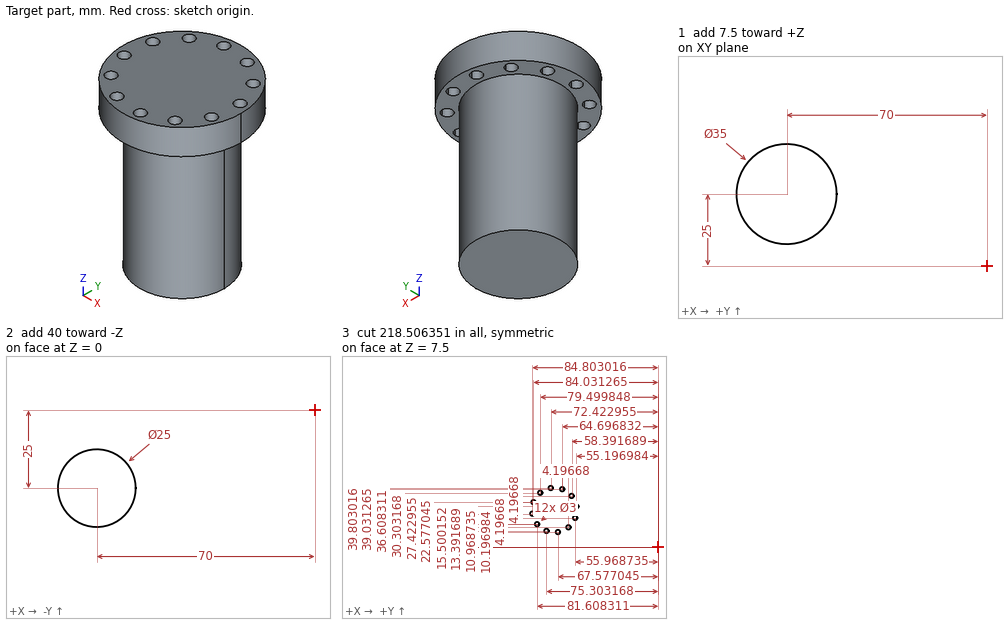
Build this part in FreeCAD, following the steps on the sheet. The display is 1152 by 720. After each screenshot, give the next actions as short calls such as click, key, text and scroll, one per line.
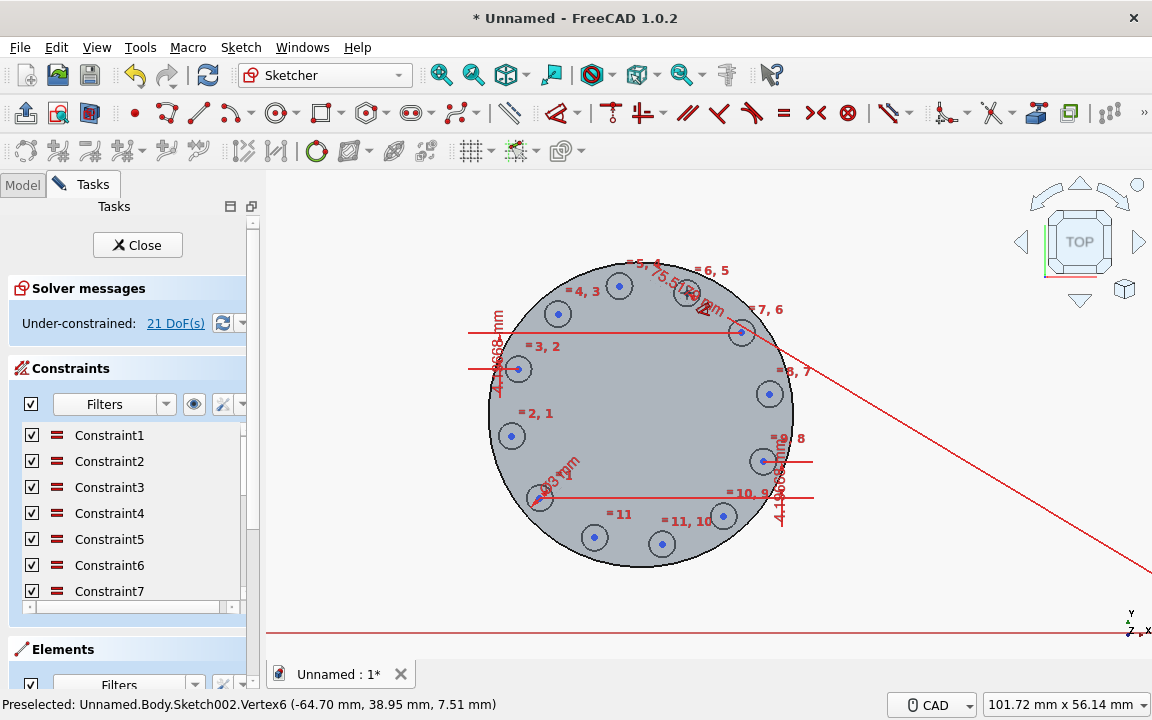
click(724, 516)
click(705, 259)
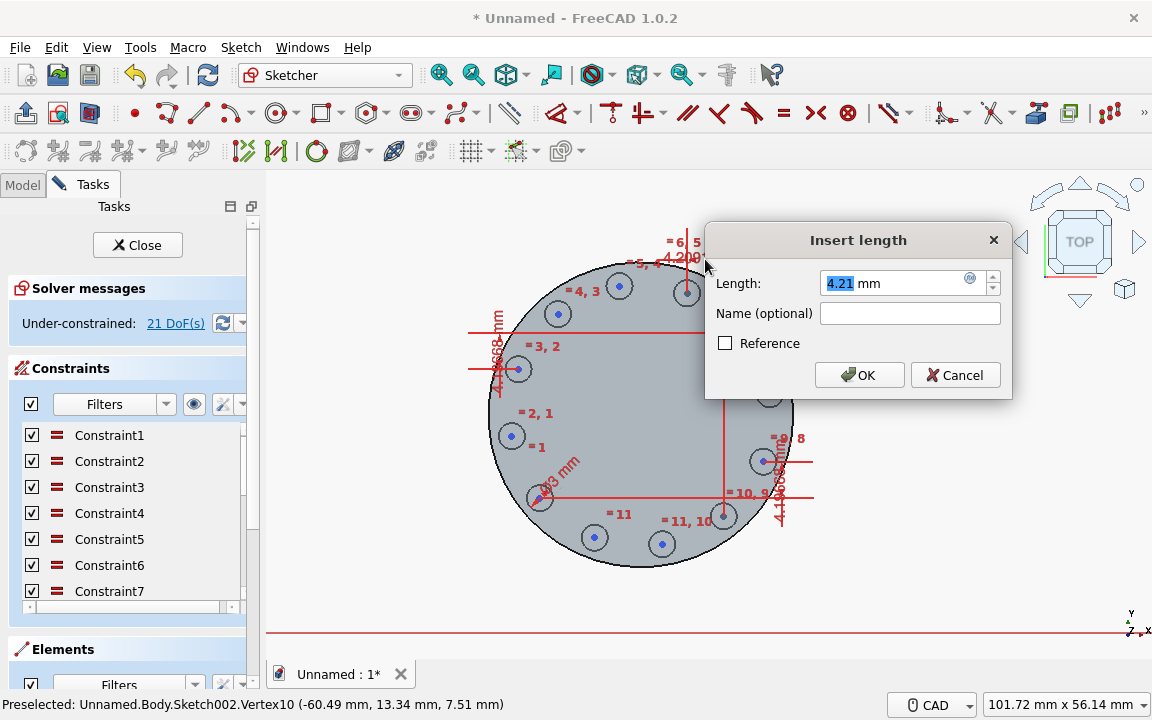
text(4.19668)
key(Return)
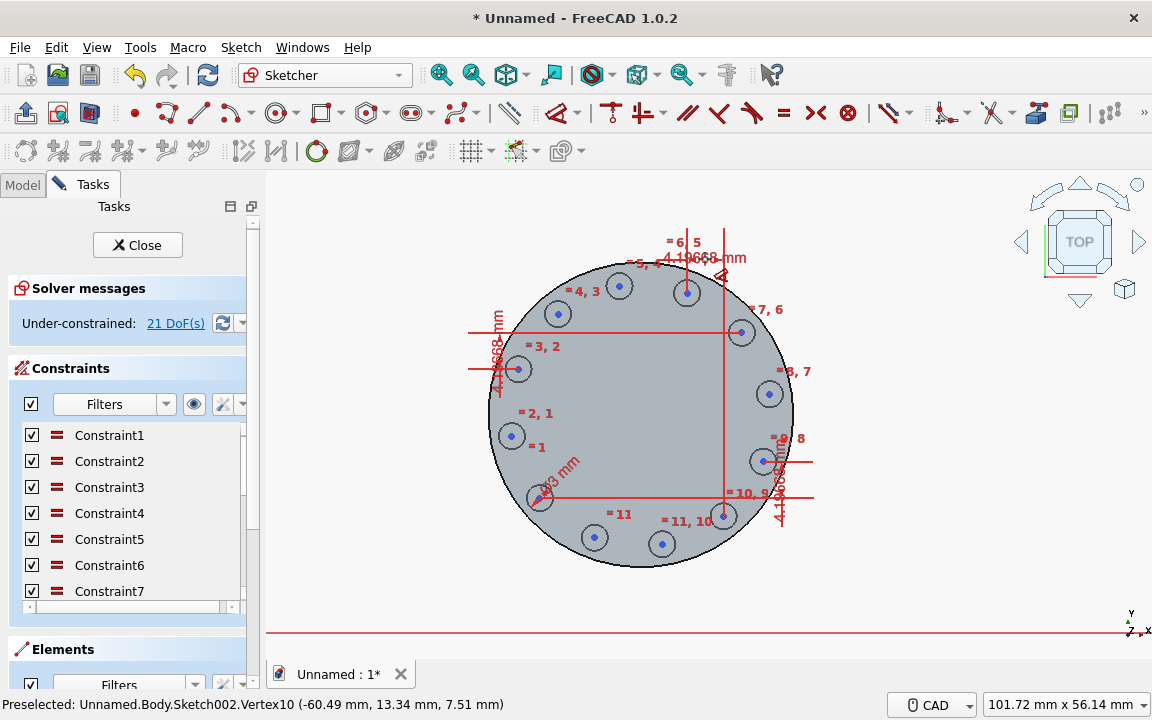
click(540, 498)
click(661, 464)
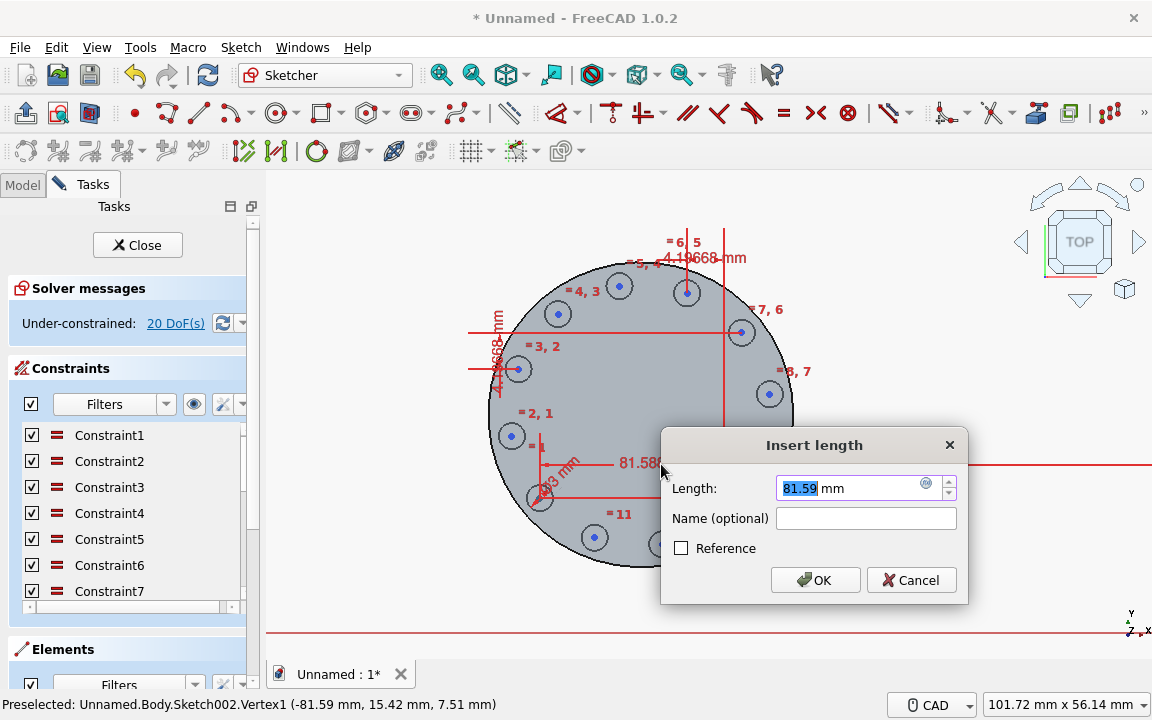
text(81.608311)
key(Return)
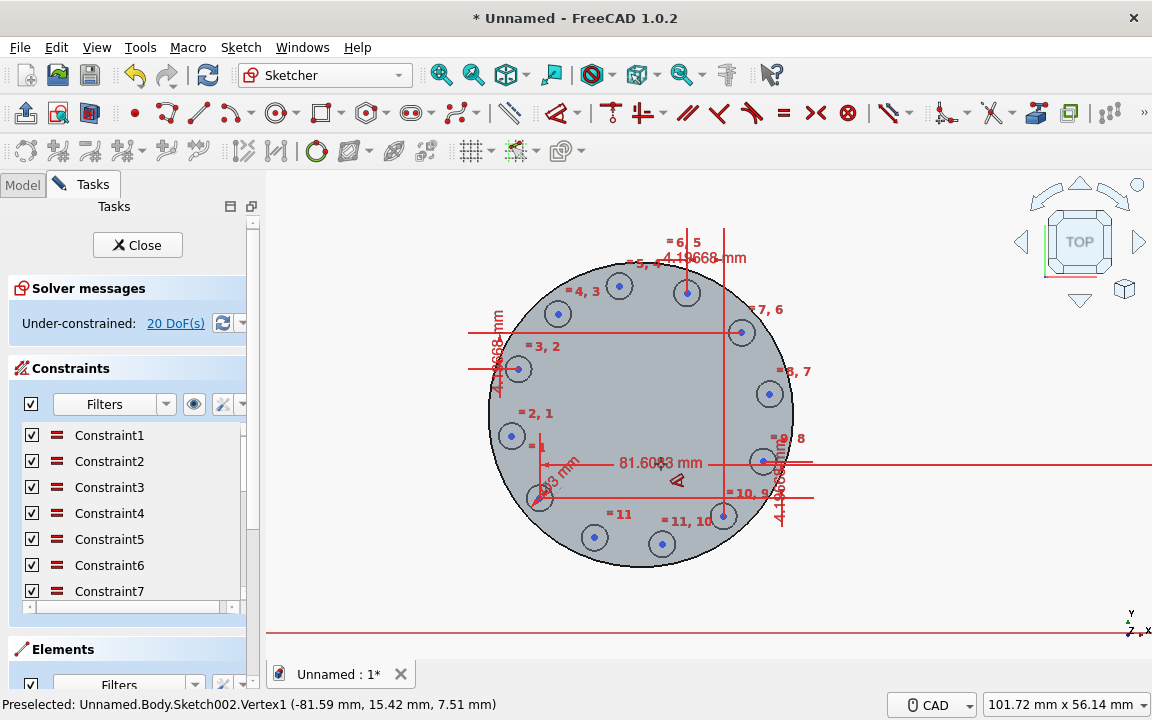
click(540, 498)
click(506, 565)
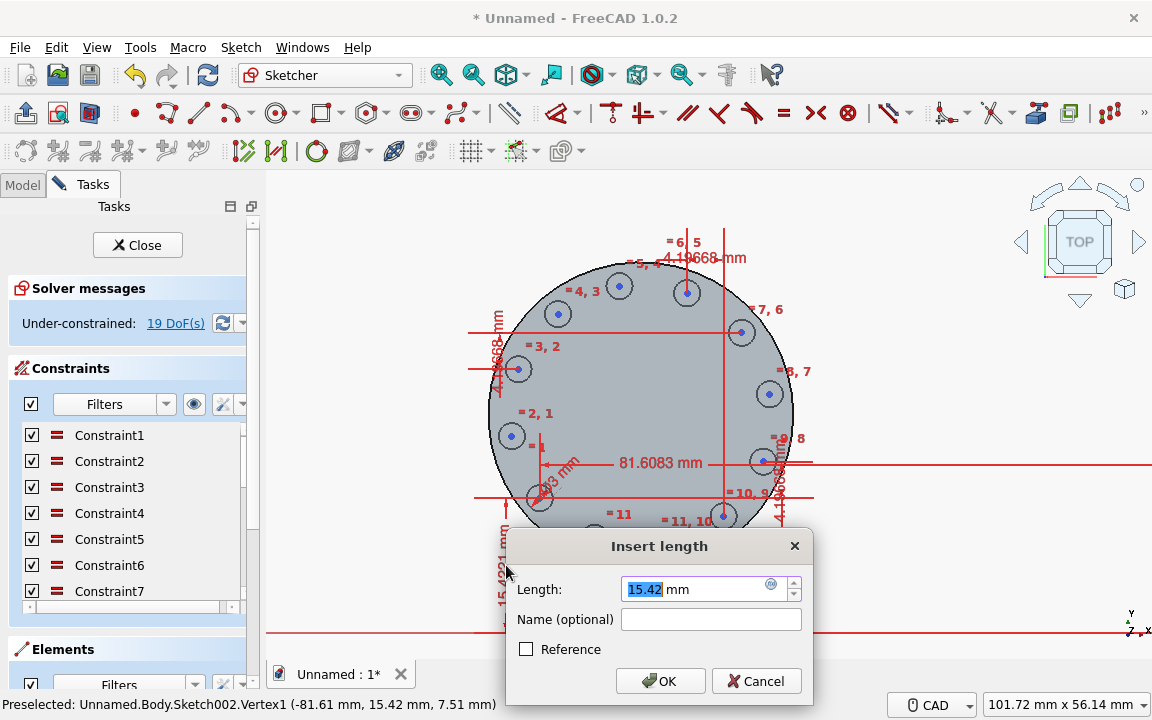
text(15.500152)
key(Return)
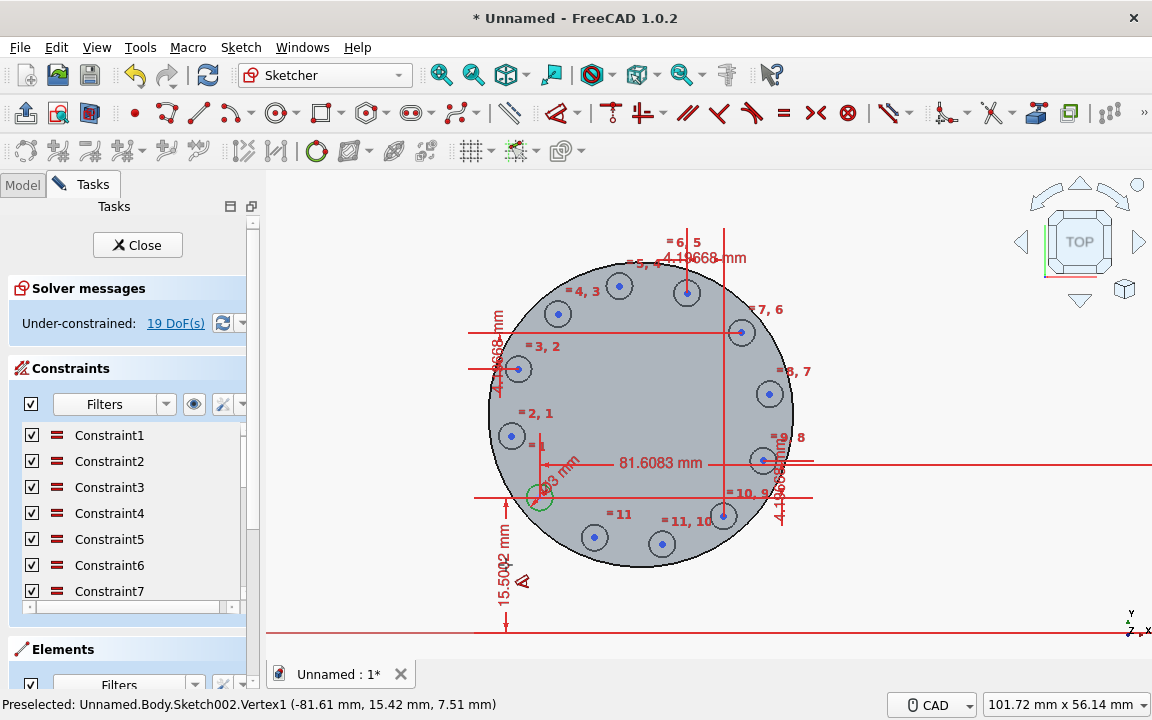
click(512, 436)
click(640, 402)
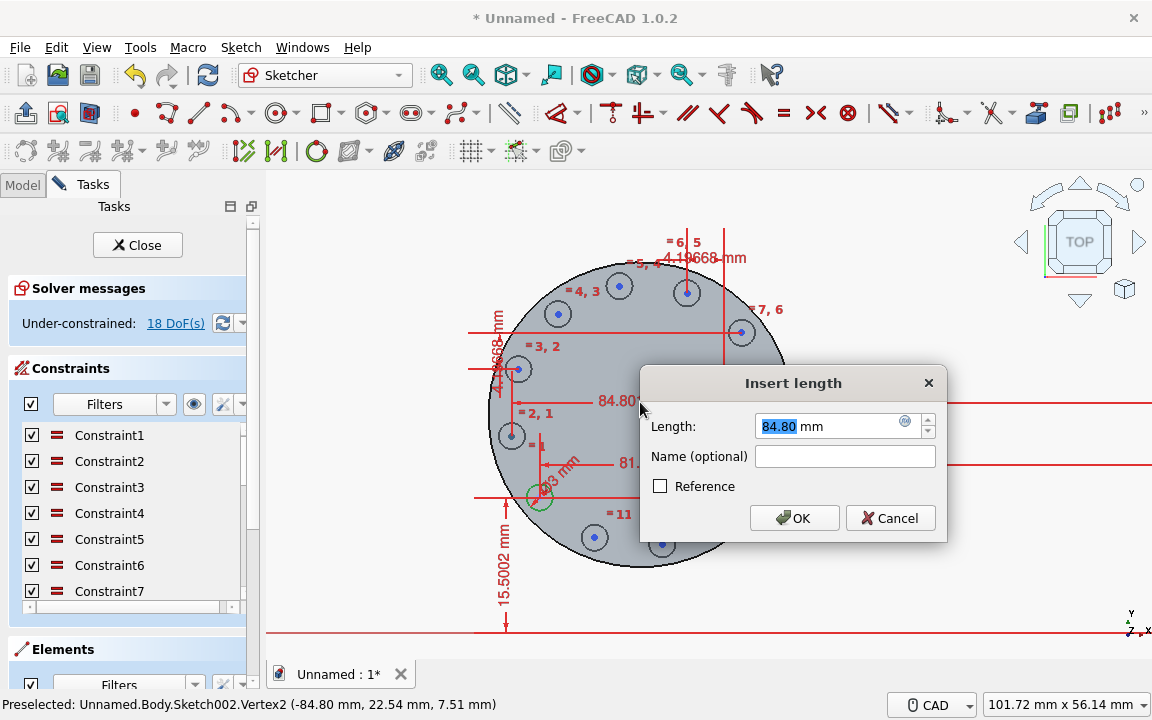
text(84.803016)
key(Return)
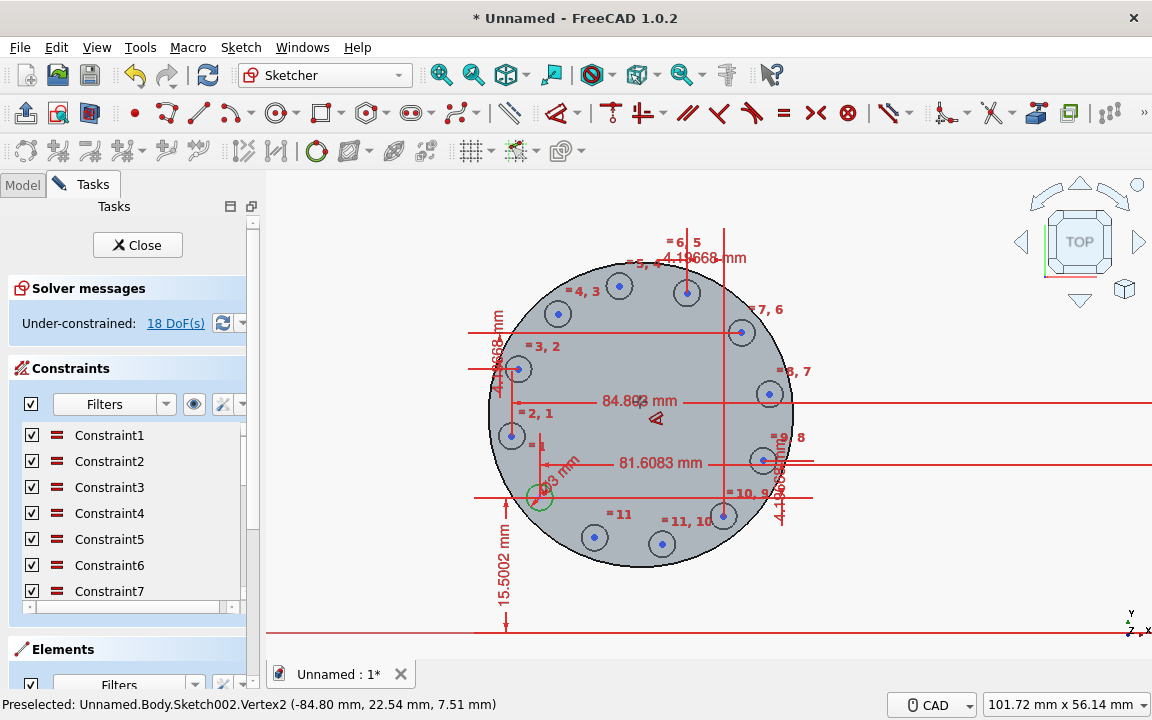
click(512, 436)
click(478, 534)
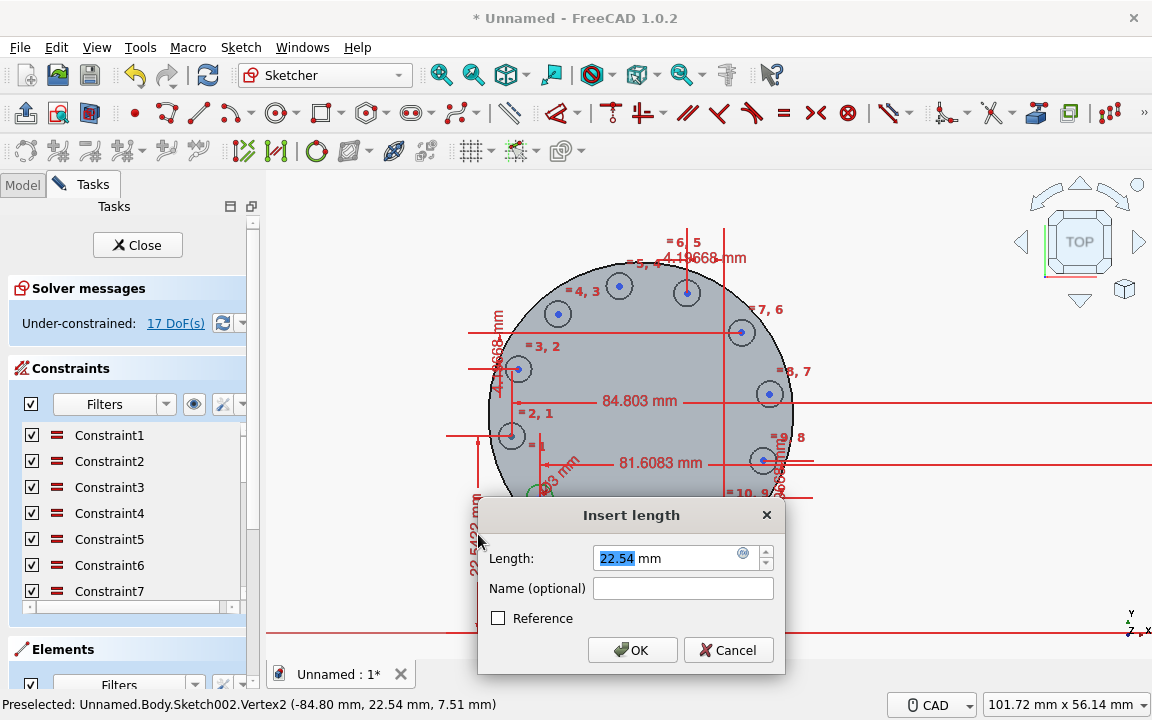
text(22.577045)
key(Return)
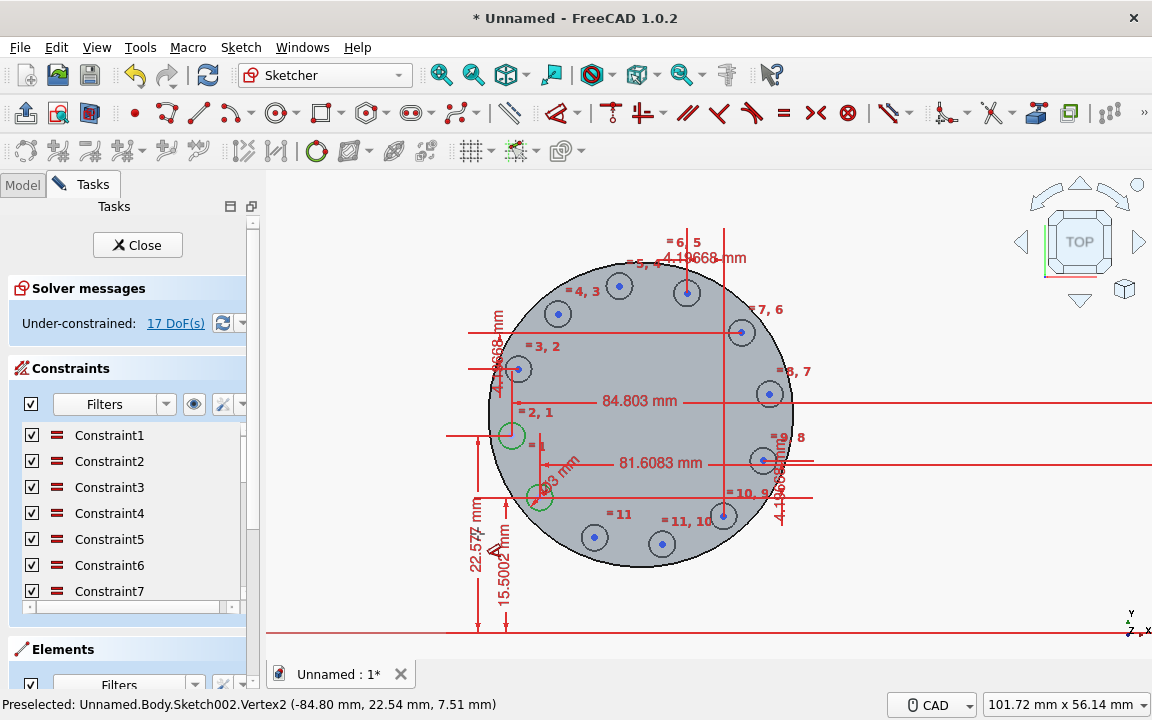
click(519, 369)
click(645, 335)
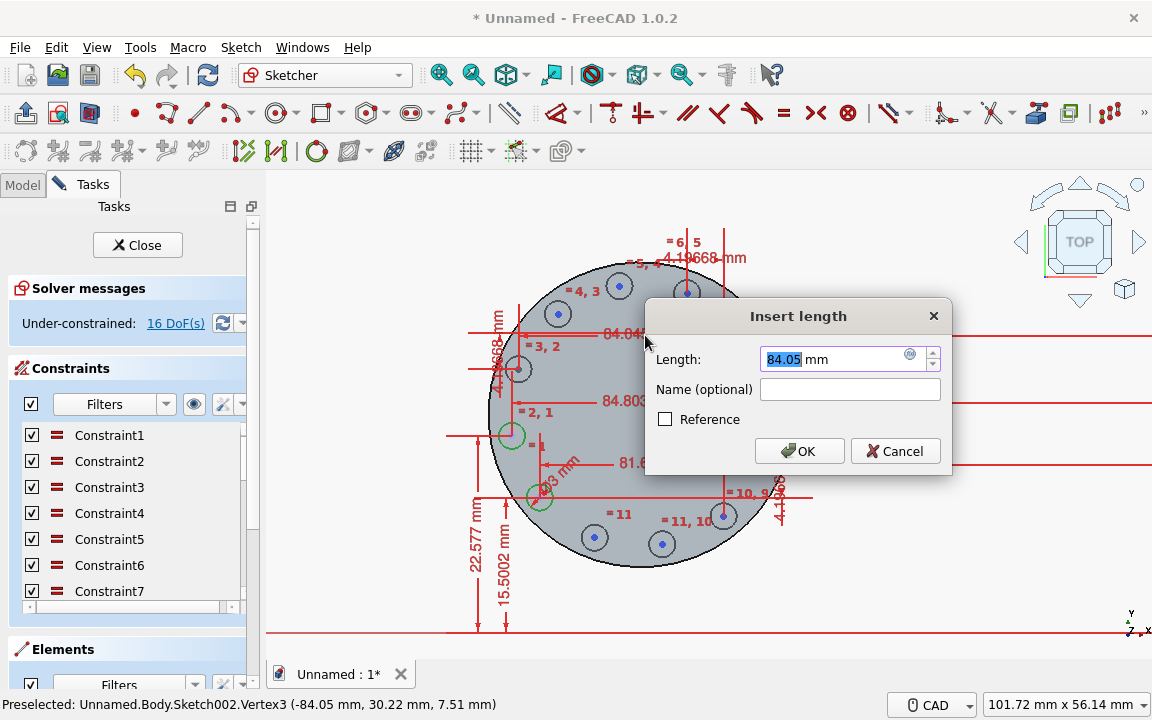
text(84.031265)
key(Return)